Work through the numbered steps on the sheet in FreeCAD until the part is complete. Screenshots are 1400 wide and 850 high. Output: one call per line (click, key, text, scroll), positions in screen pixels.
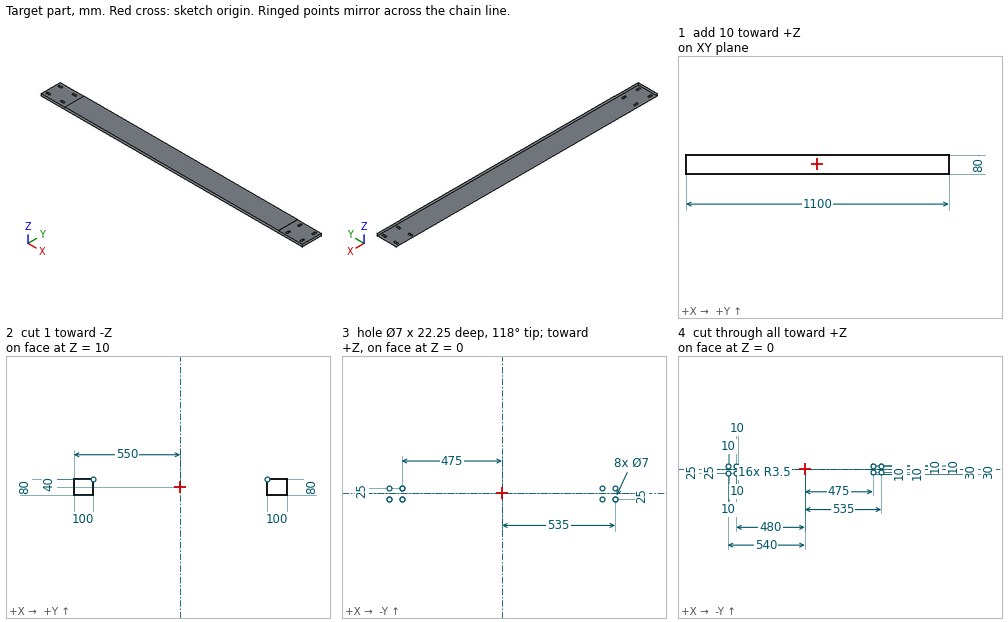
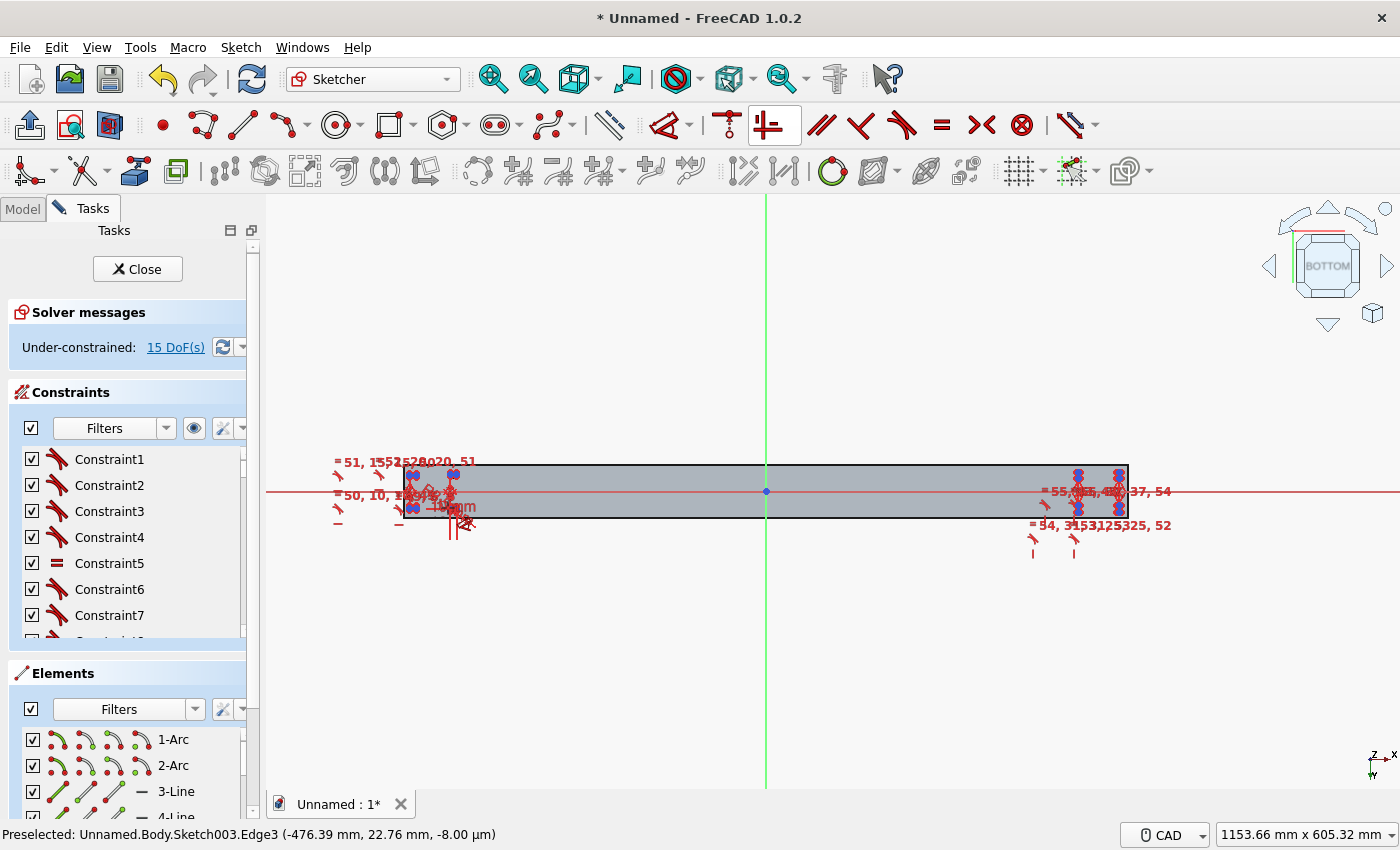
scroll(412, 506, up, 10)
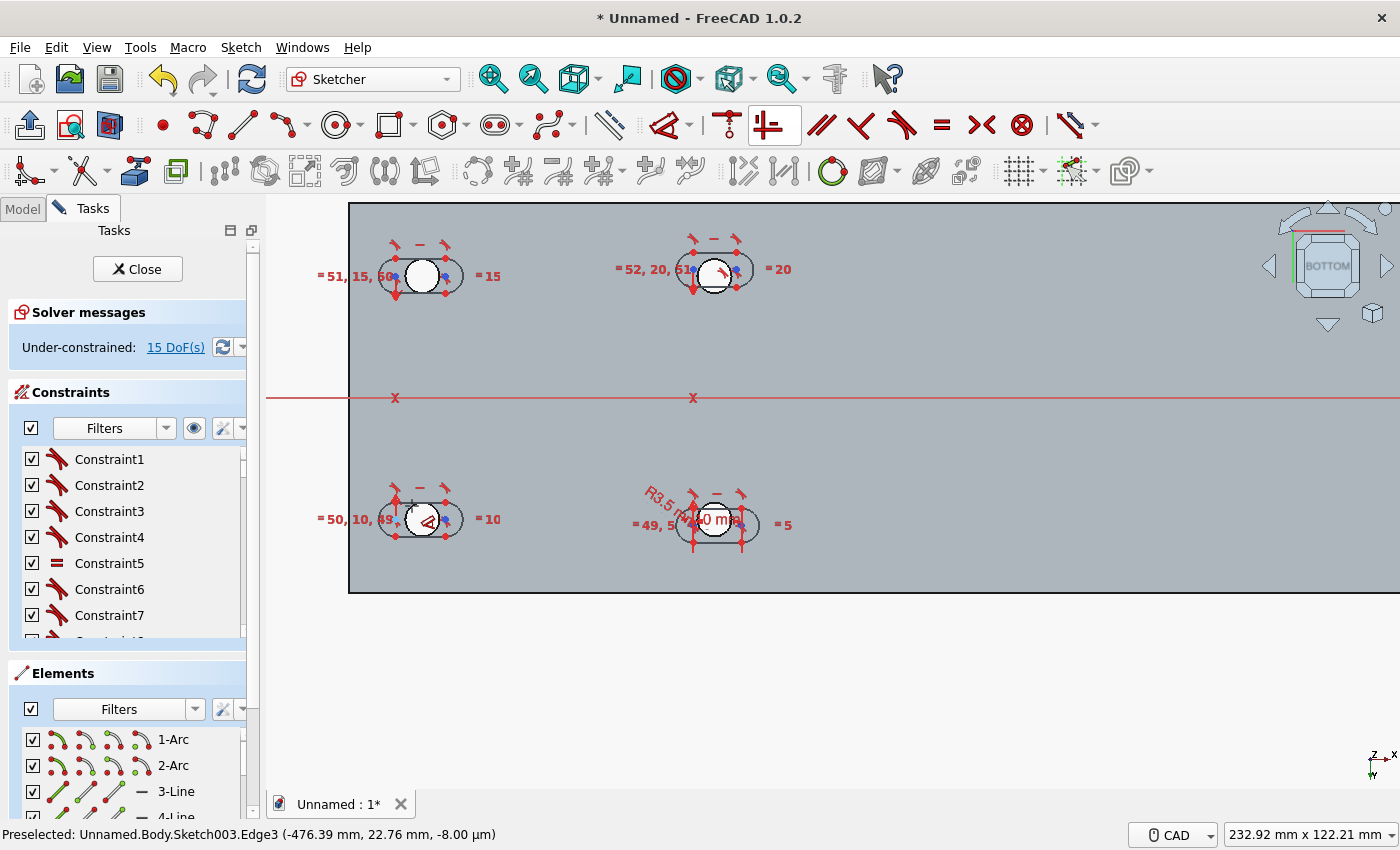
click(411, 503)
click(421, 469)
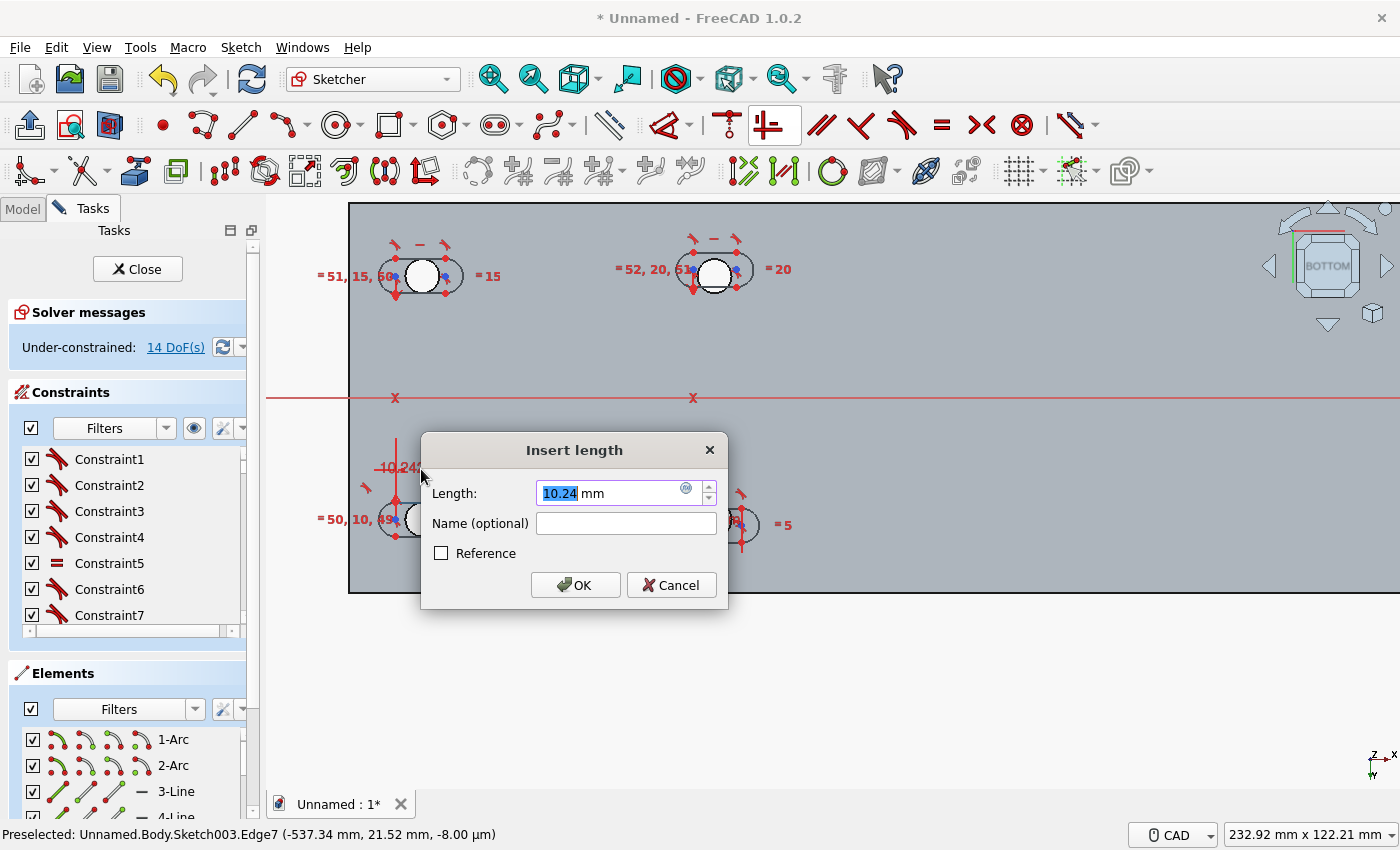
text(10)
key(Return)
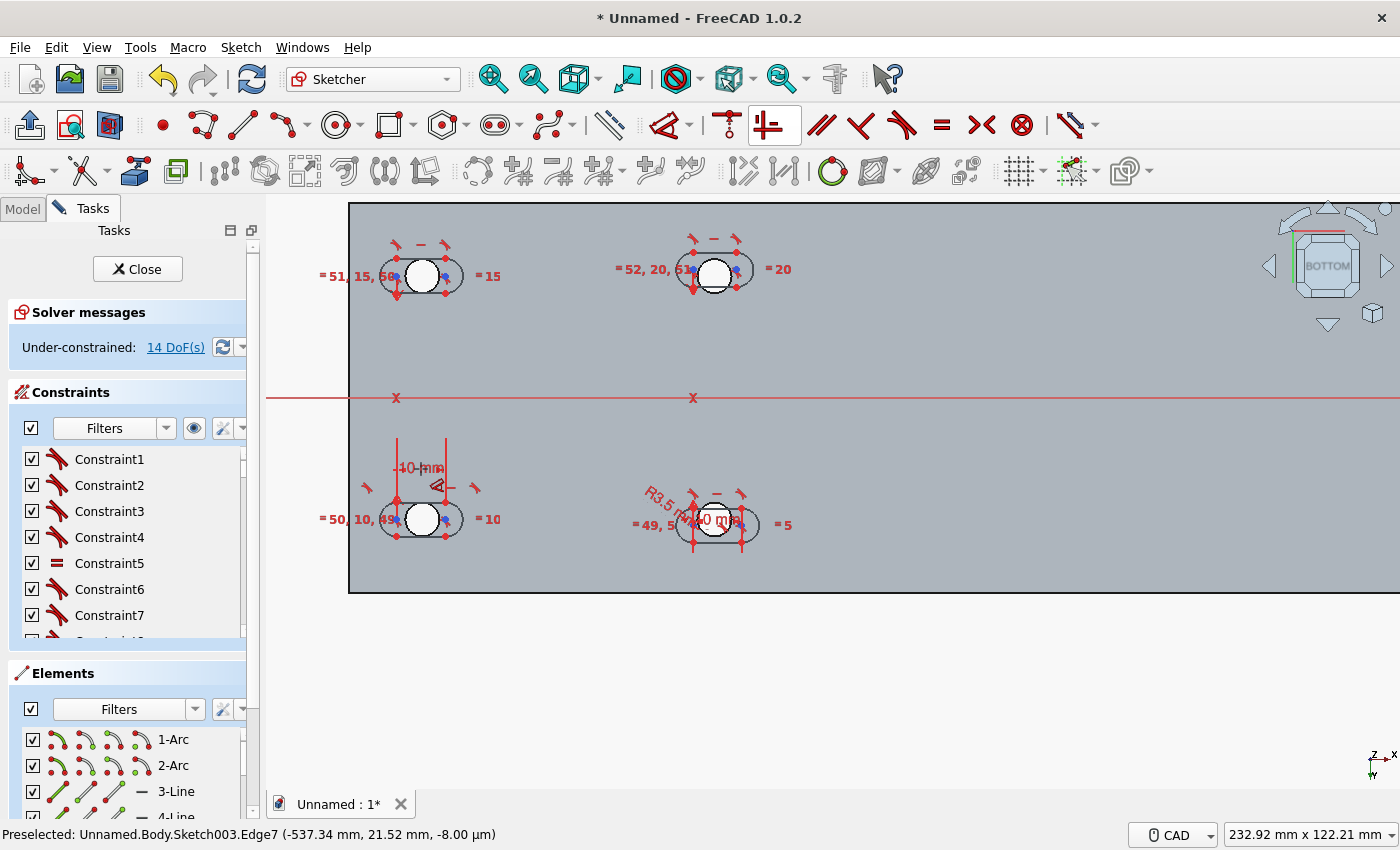
click(412, 259)
click(421, 225)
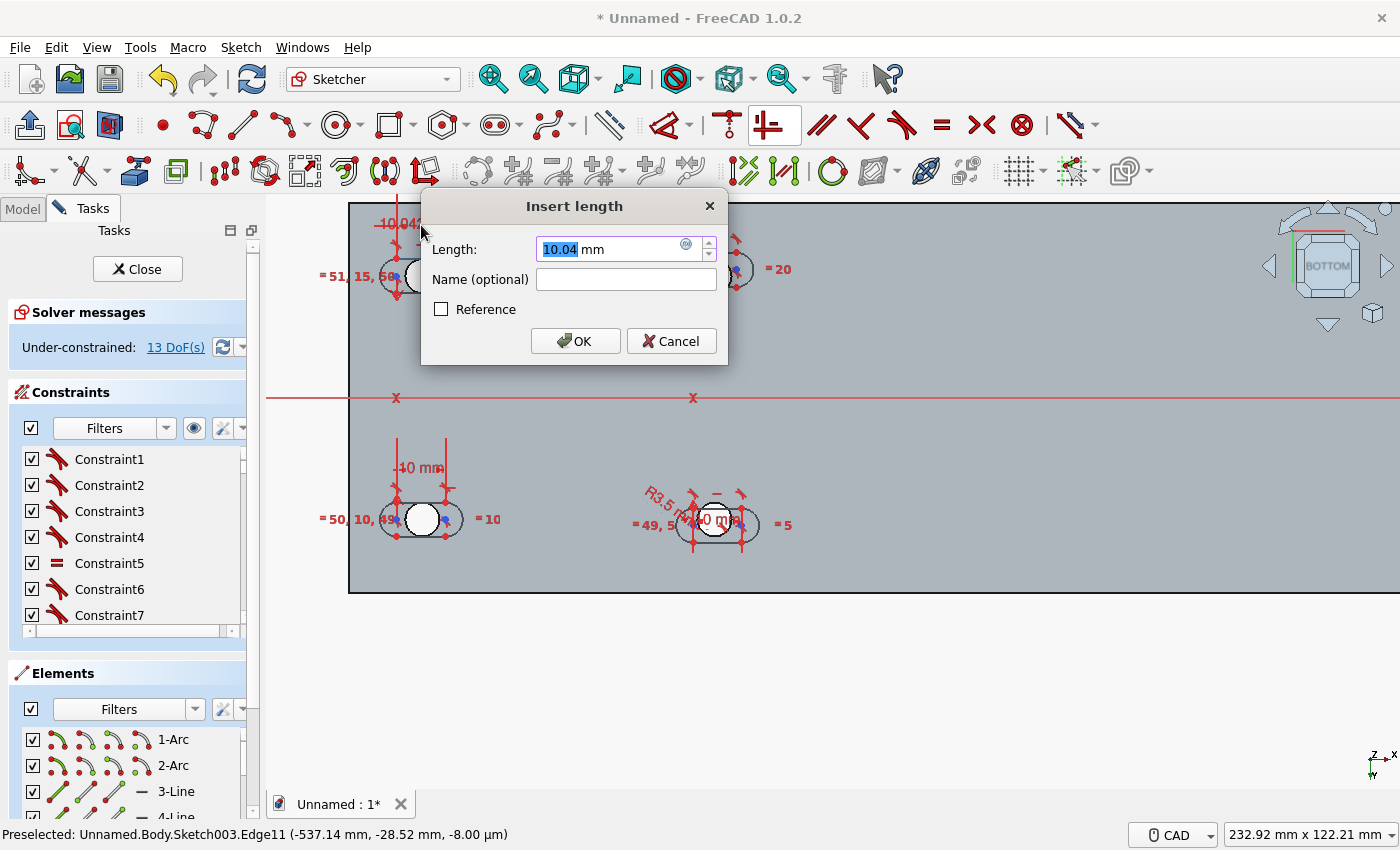
text(10)
key(Return)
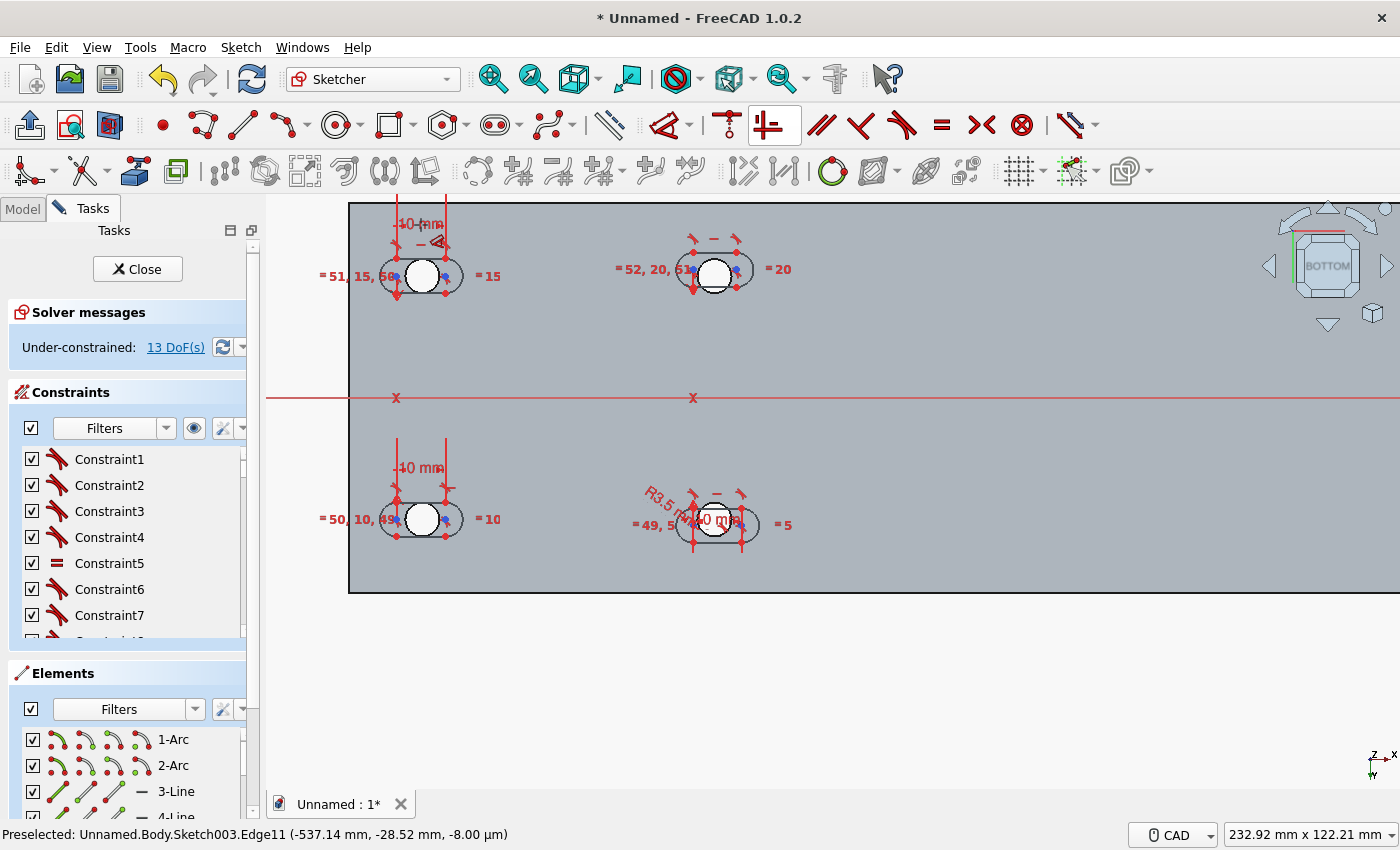
click(706, 253)
click(715, 311)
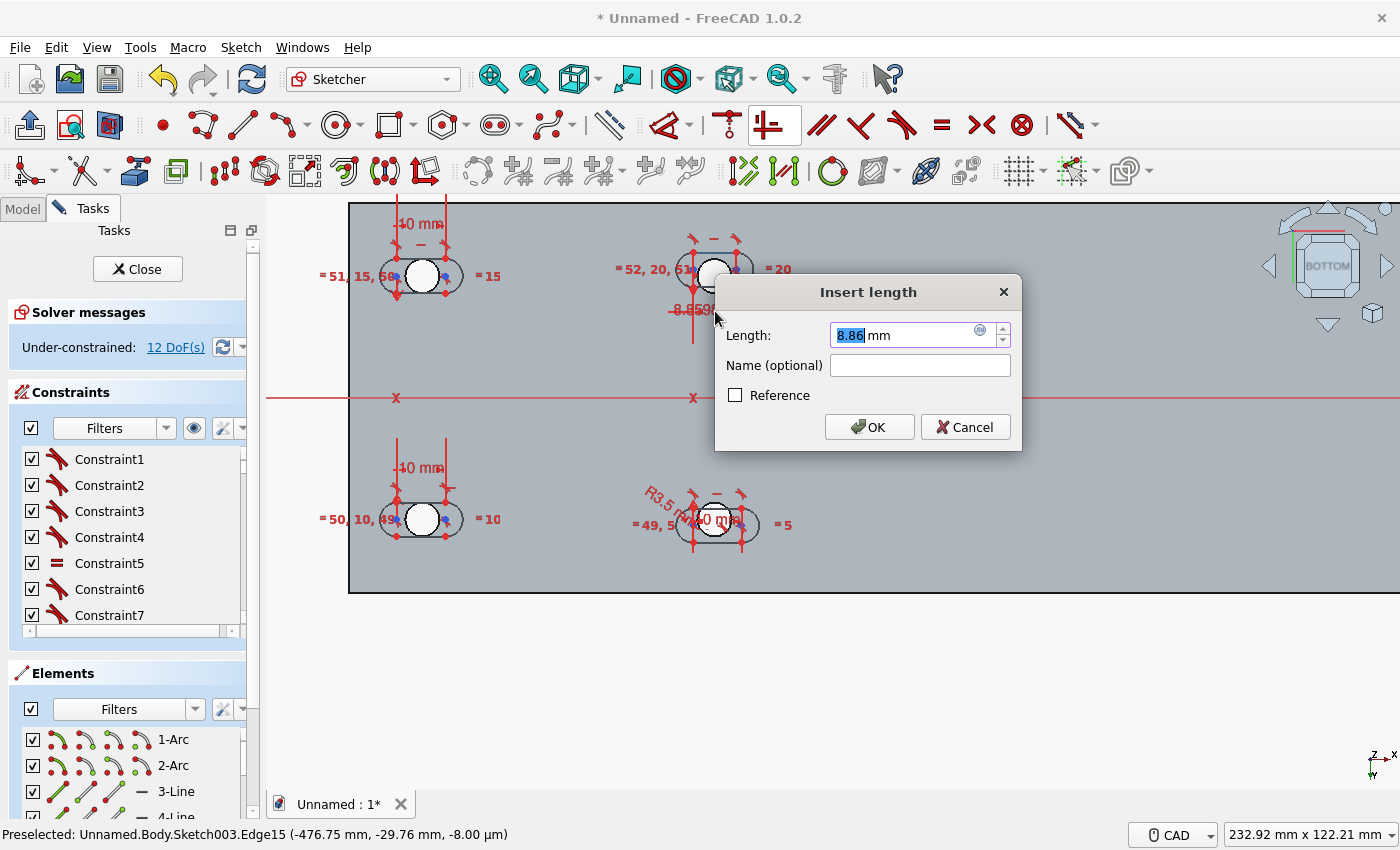
text(10)
key(Return)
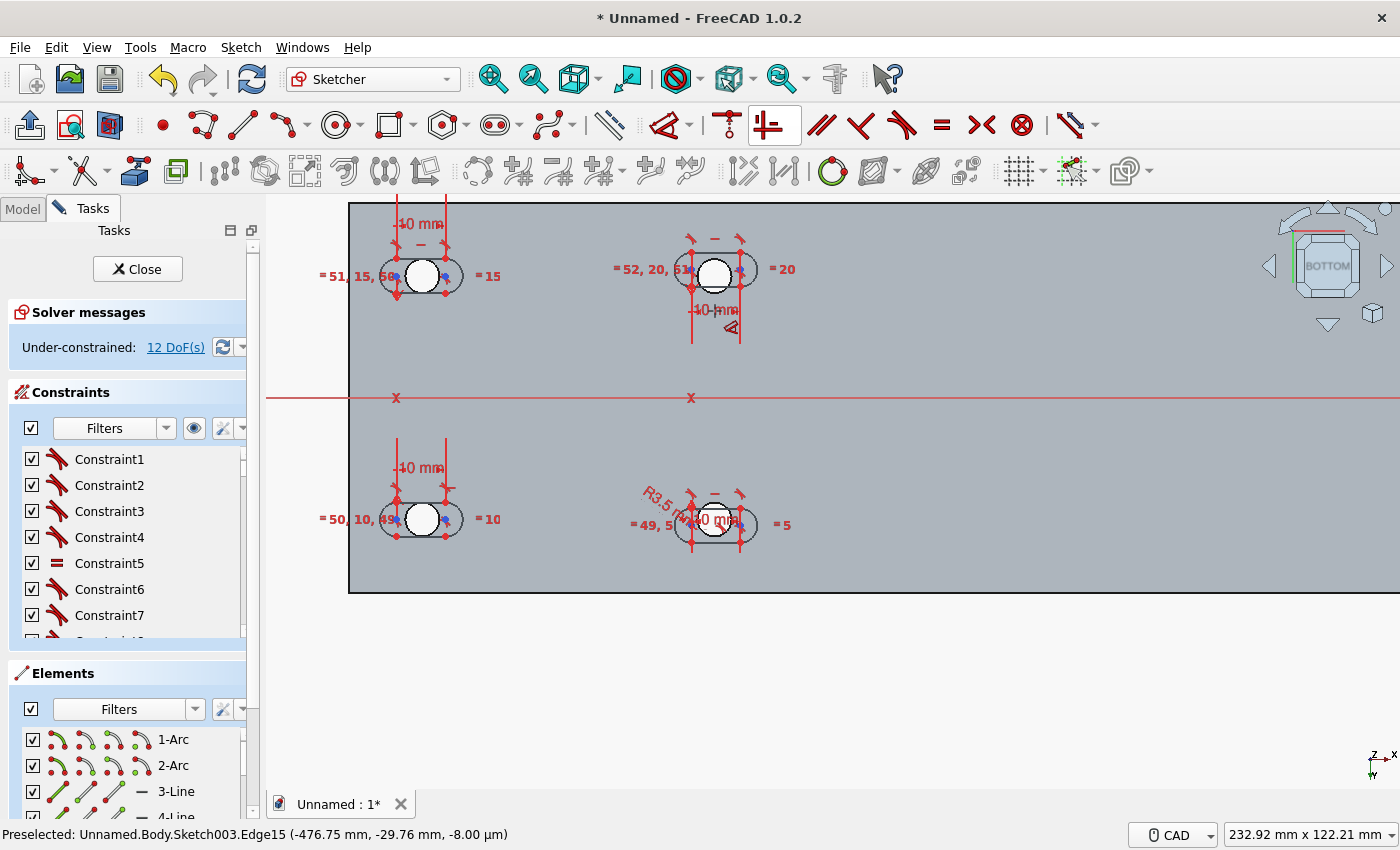
scroll(412, 506, down, 10)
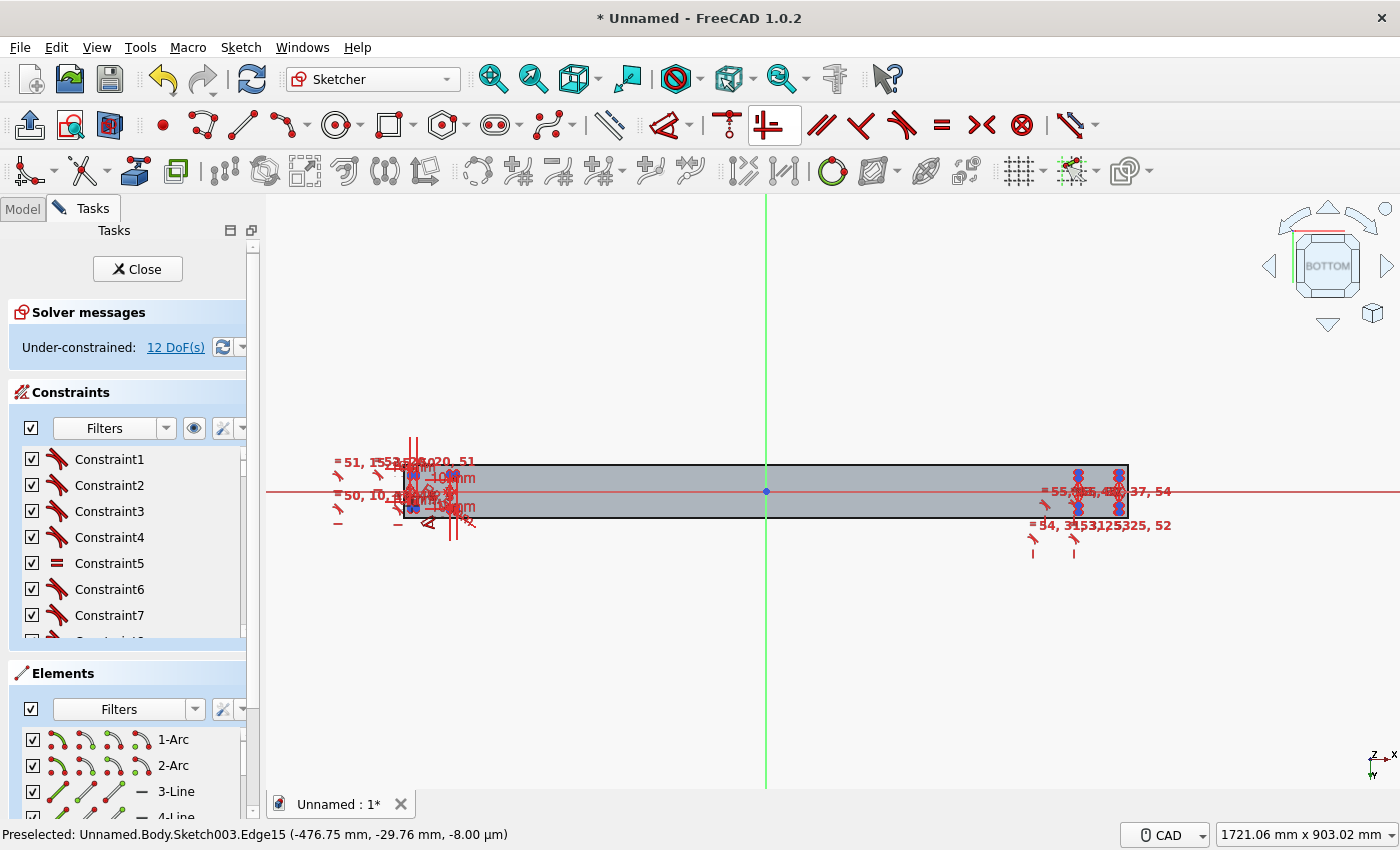
scroll(1117, 510, up, 10)